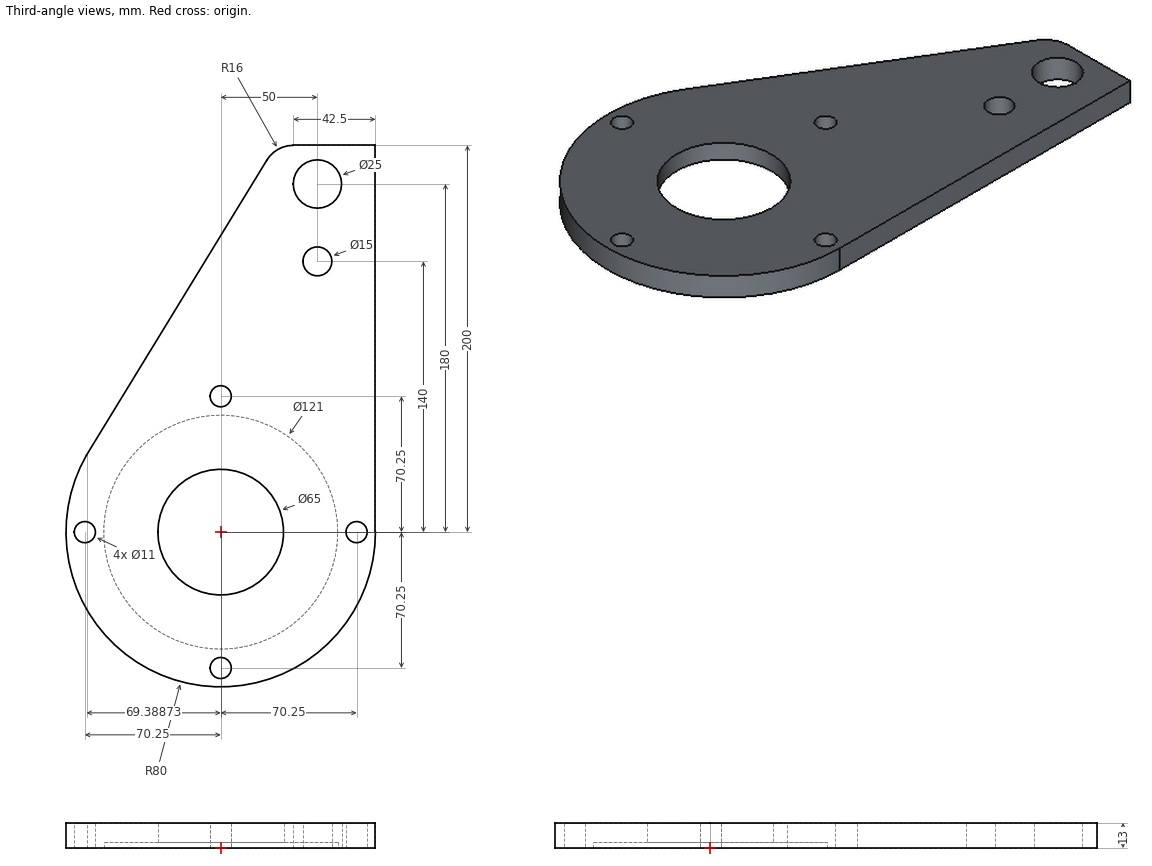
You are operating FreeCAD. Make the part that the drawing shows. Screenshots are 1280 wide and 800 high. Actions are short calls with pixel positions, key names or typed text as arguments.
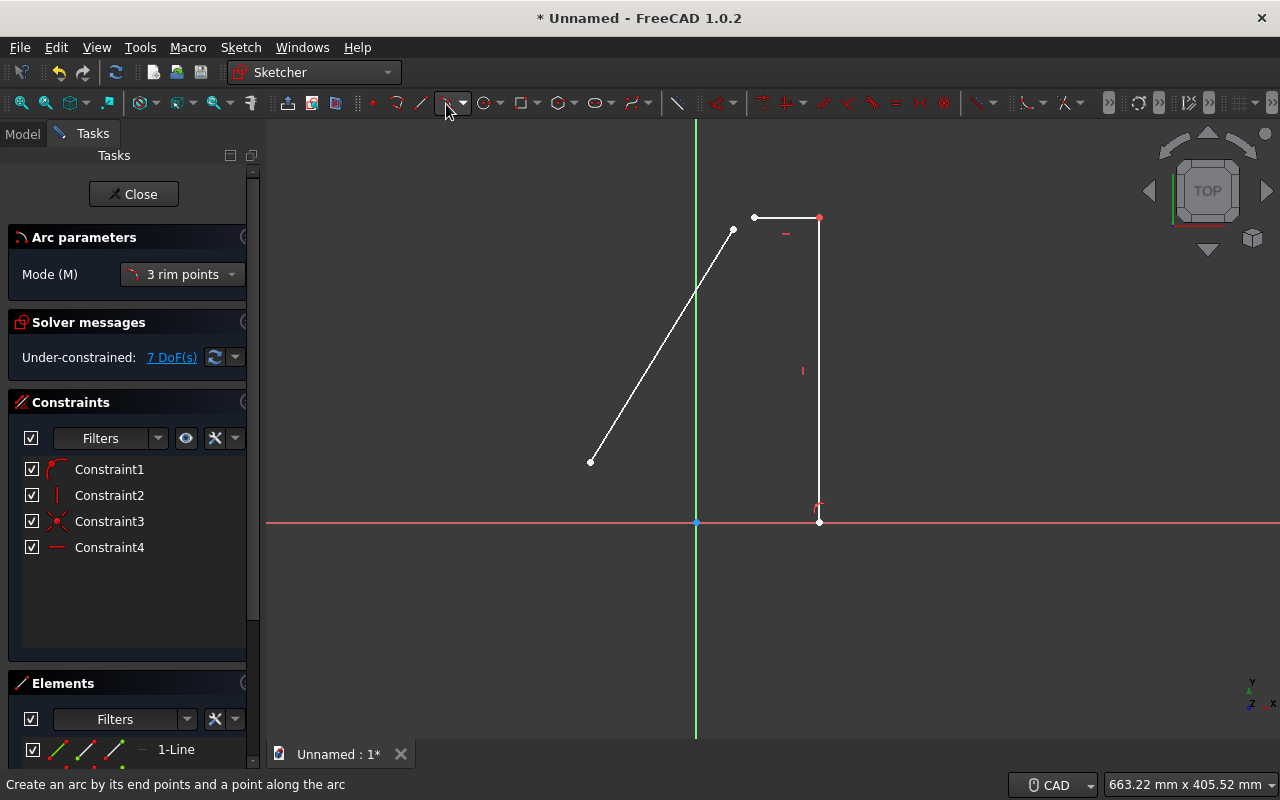
click(590, 463)
click(819, 523)
click(665, 641)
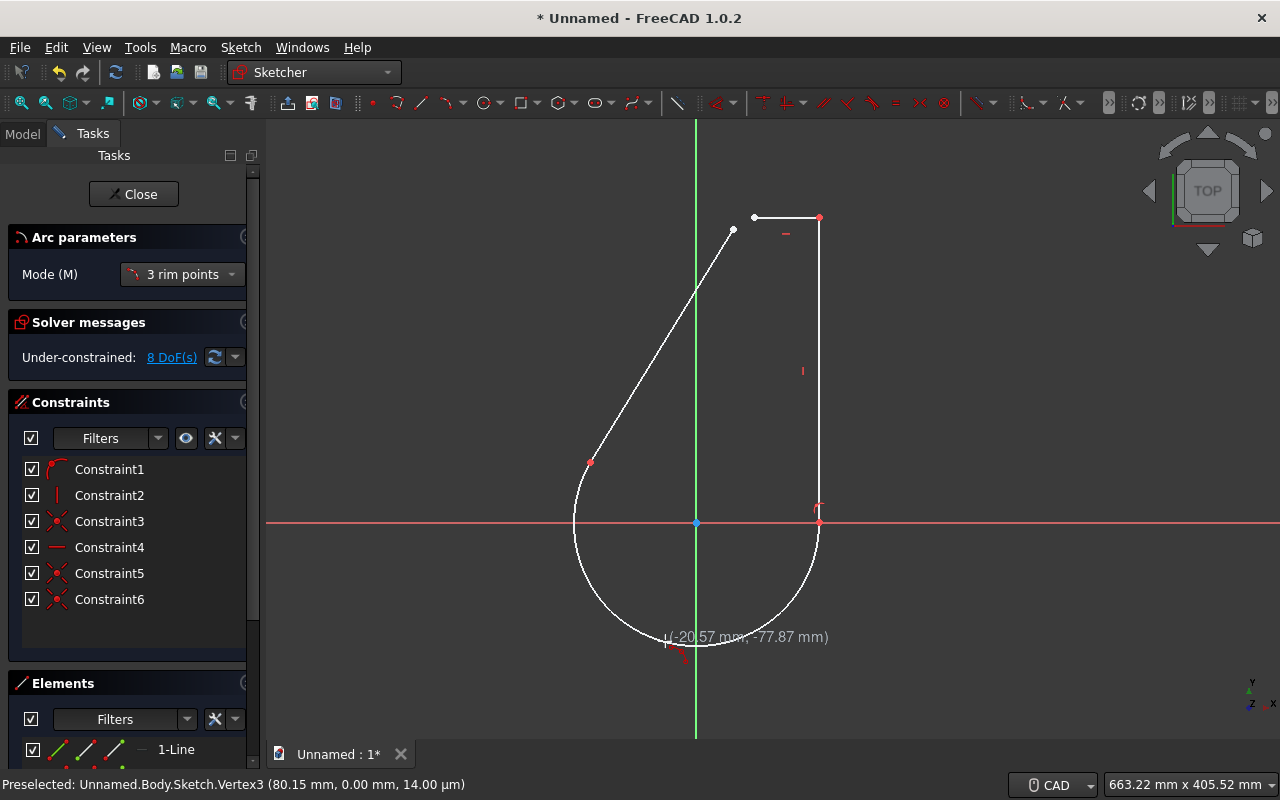
click(754, 218)
click(733, 230)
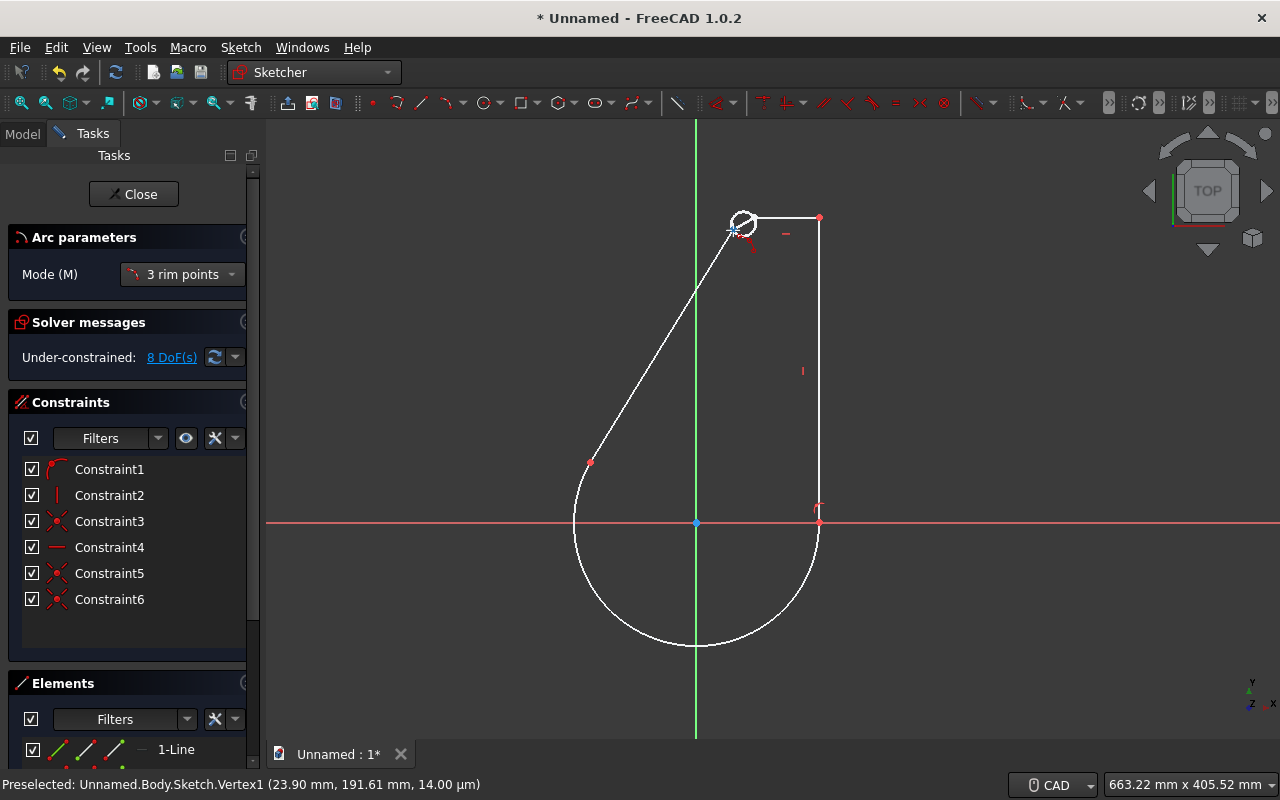
scroll(742, 220, up, 9)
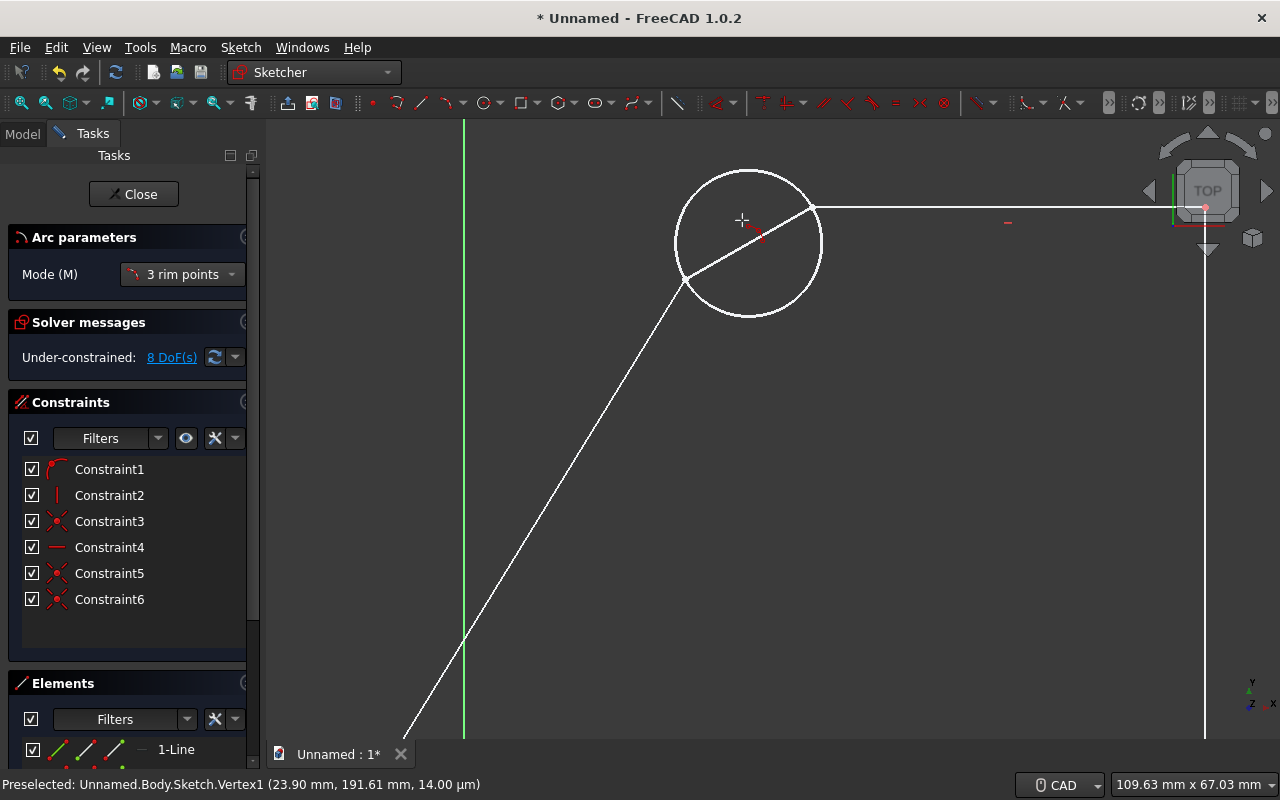
click(739, 221)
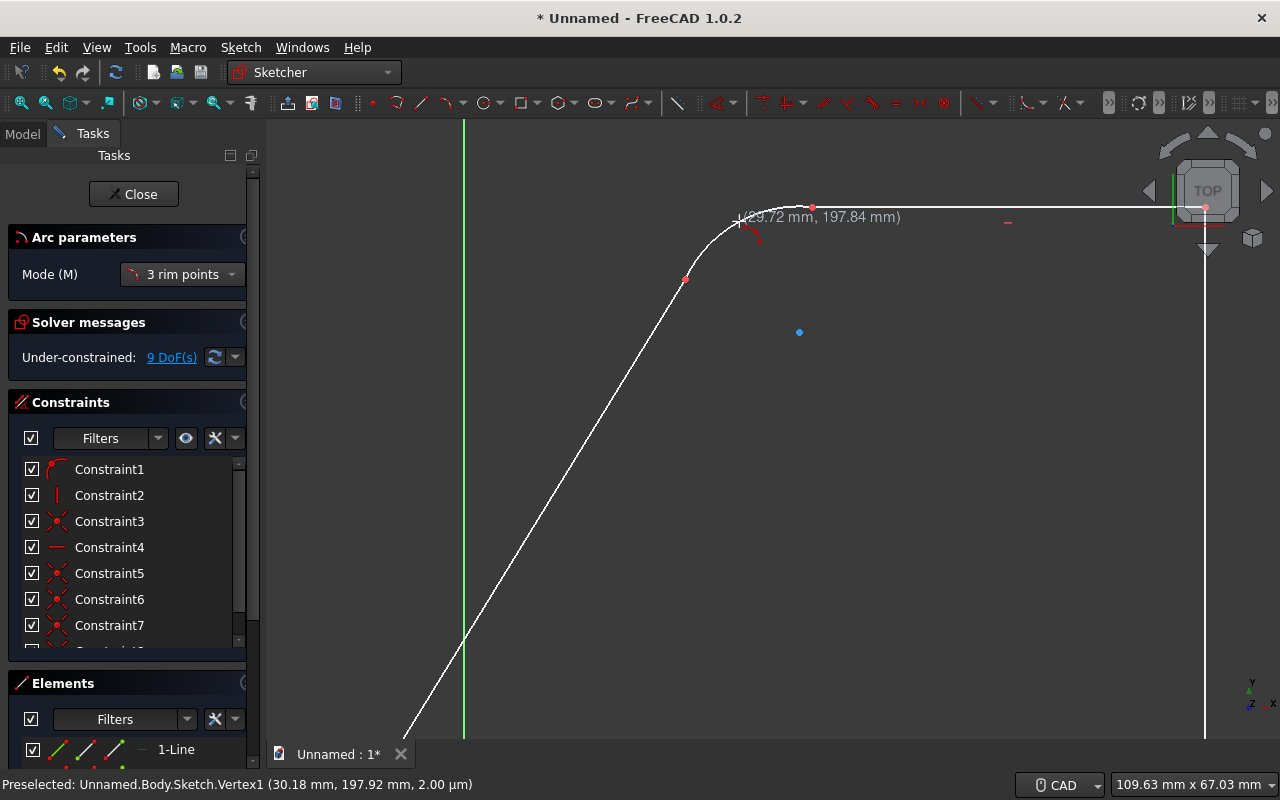
key(g)
key(c)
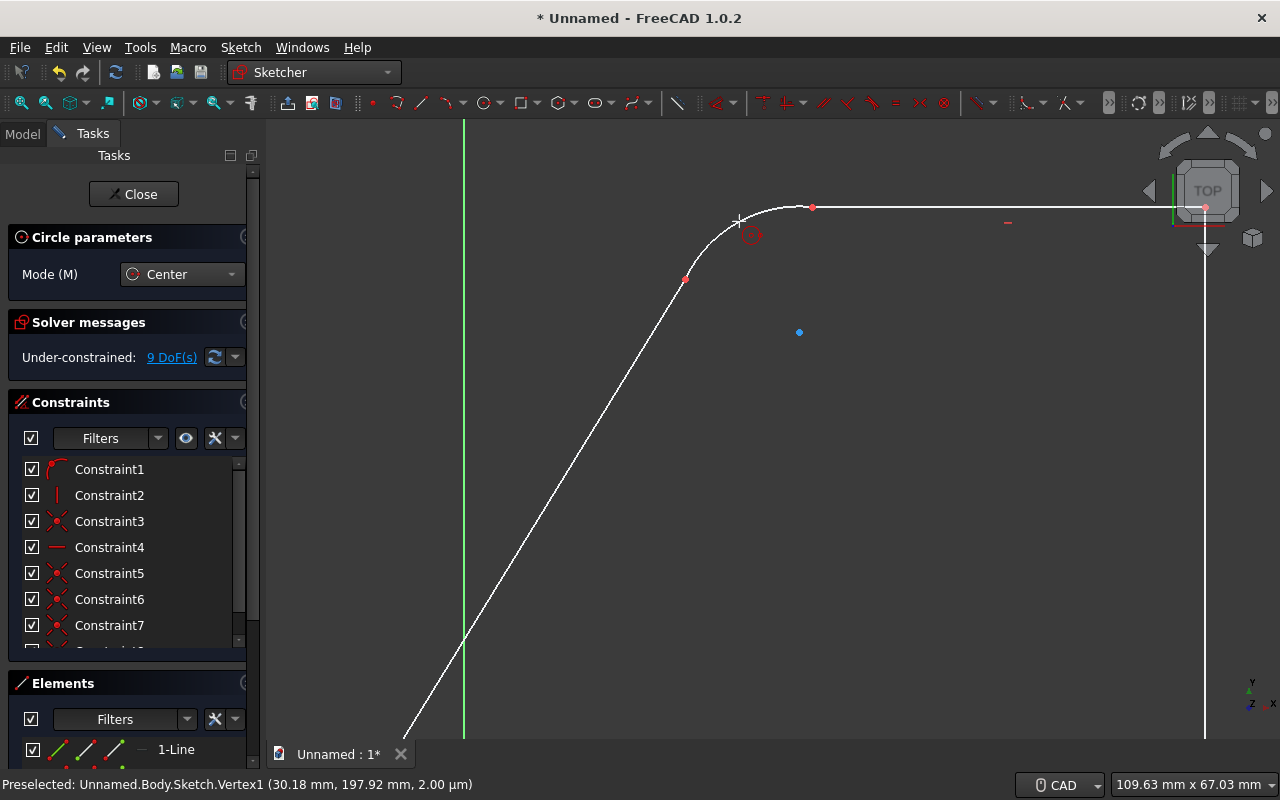
scroll(742, 220, down, 9)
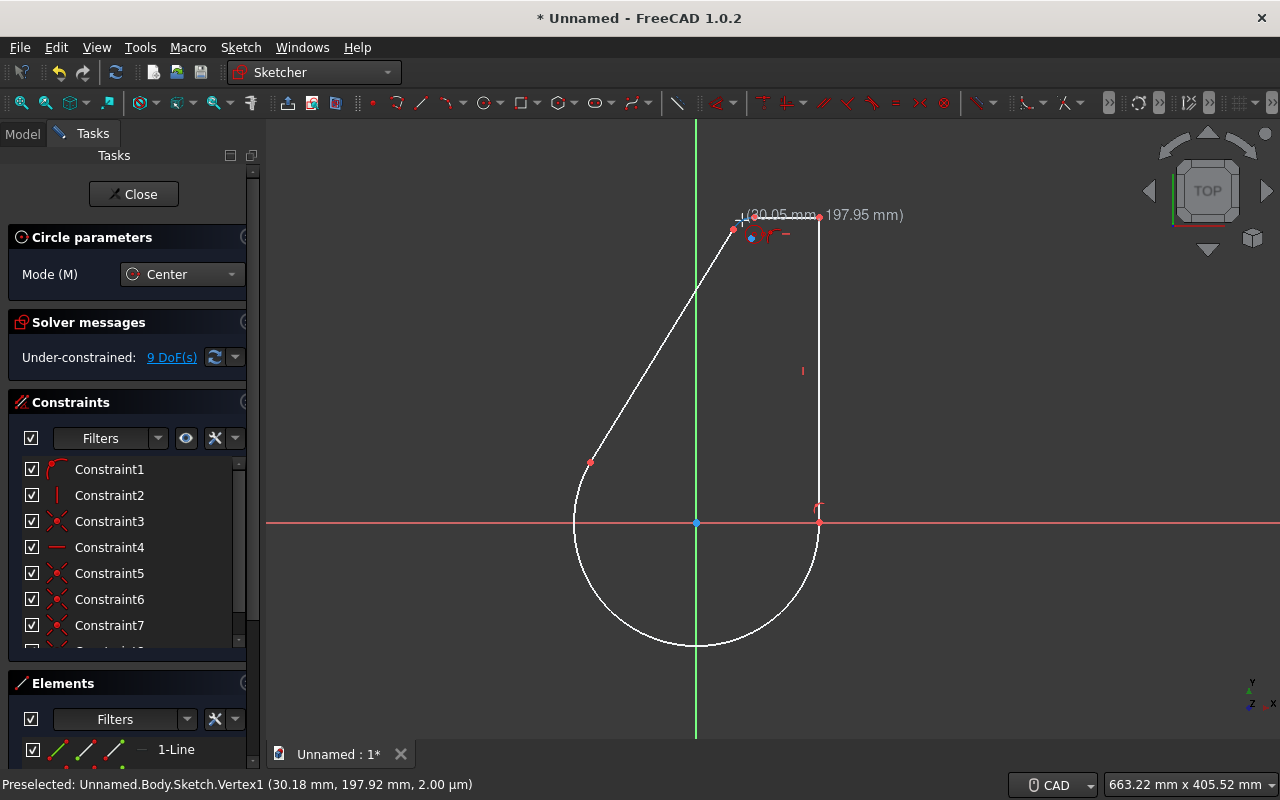
click(696, 523)
click(732, 488)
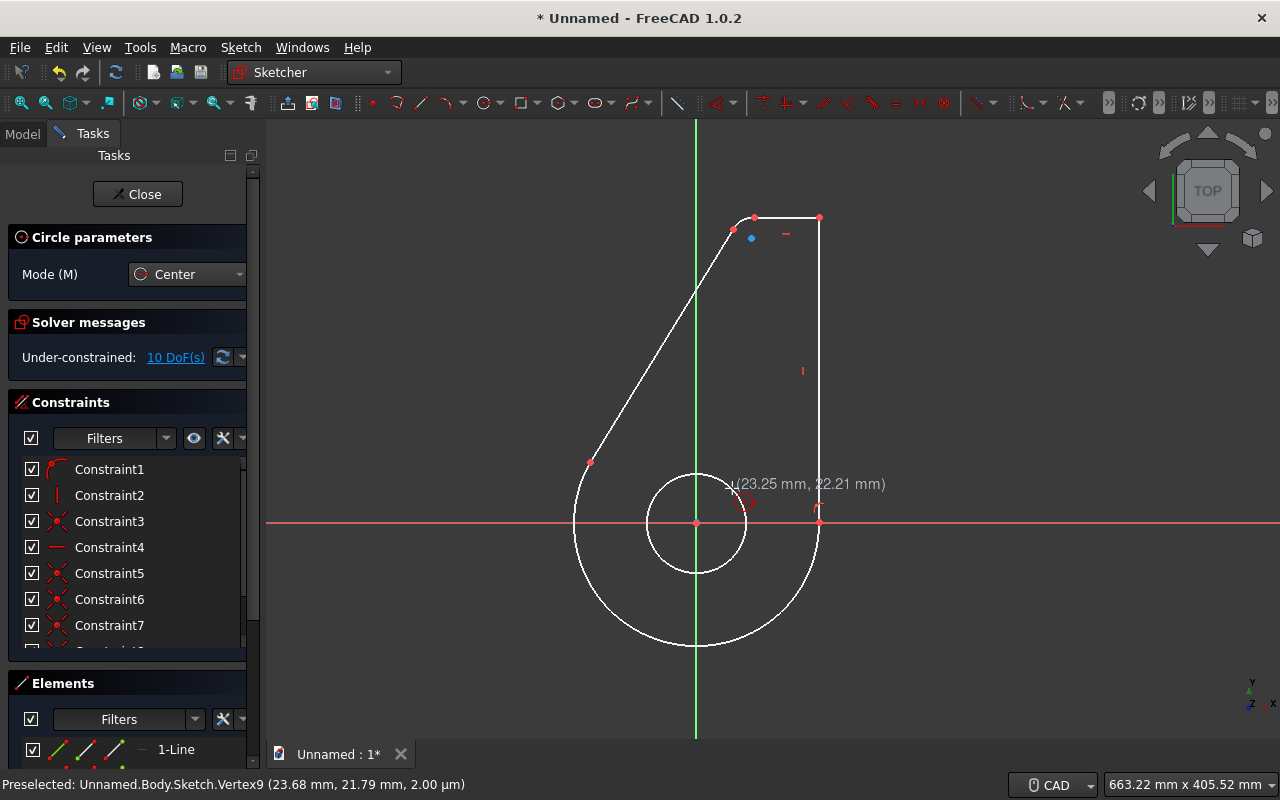
scroll(773, 309, up, 4)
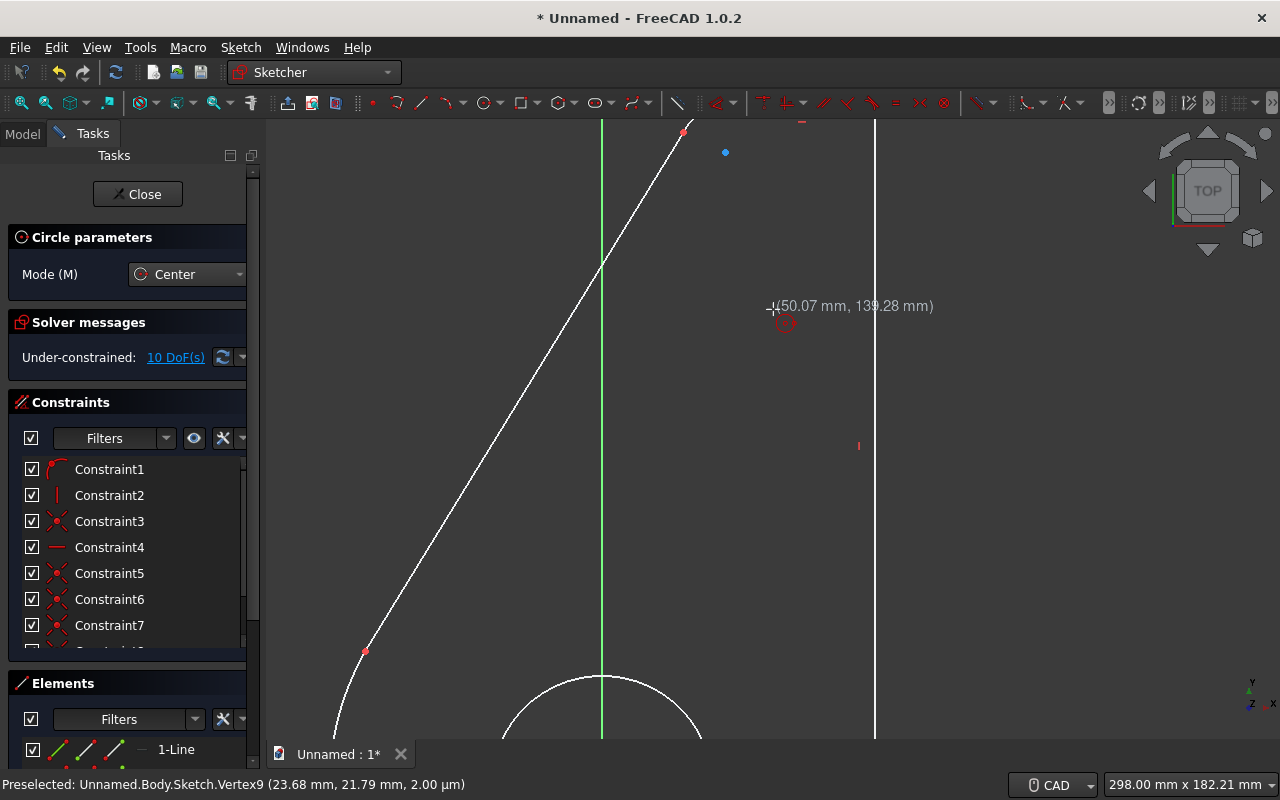
click(772, 308)
click(790, 290)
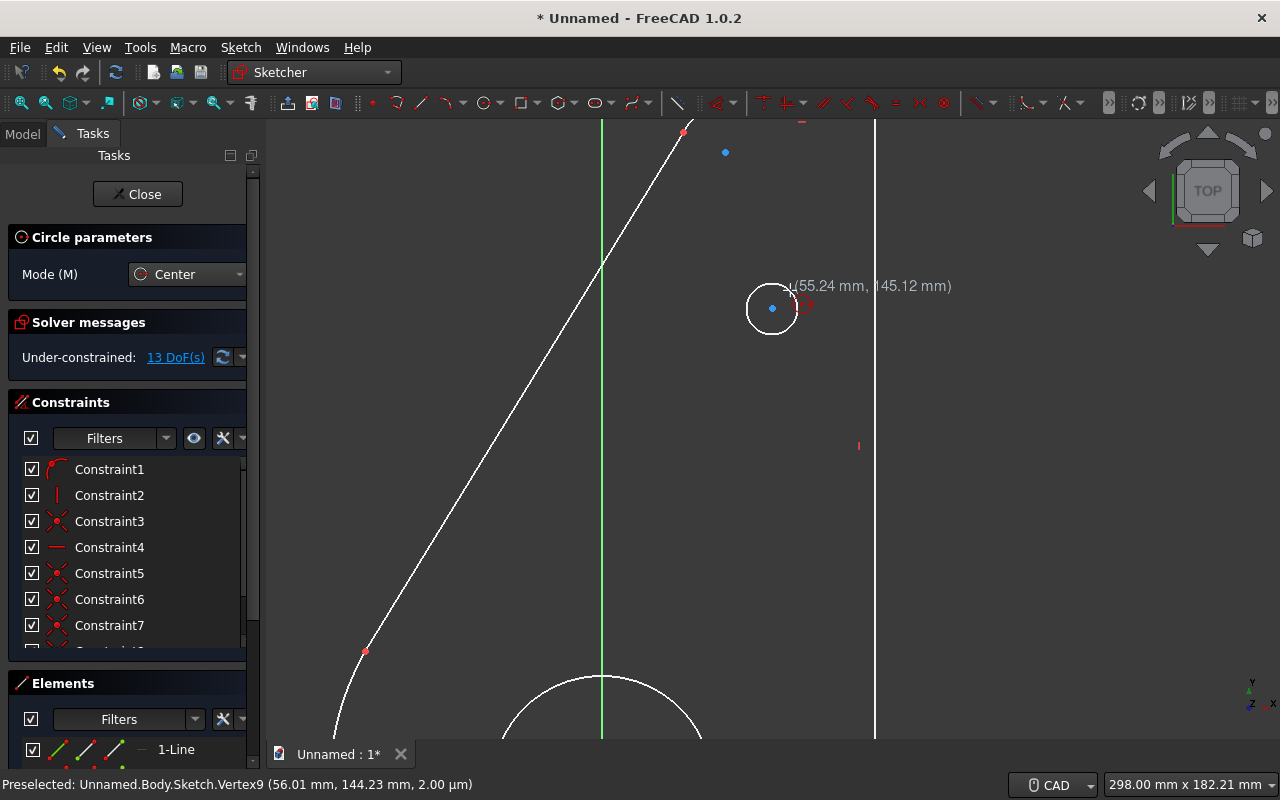
click(772, 172)